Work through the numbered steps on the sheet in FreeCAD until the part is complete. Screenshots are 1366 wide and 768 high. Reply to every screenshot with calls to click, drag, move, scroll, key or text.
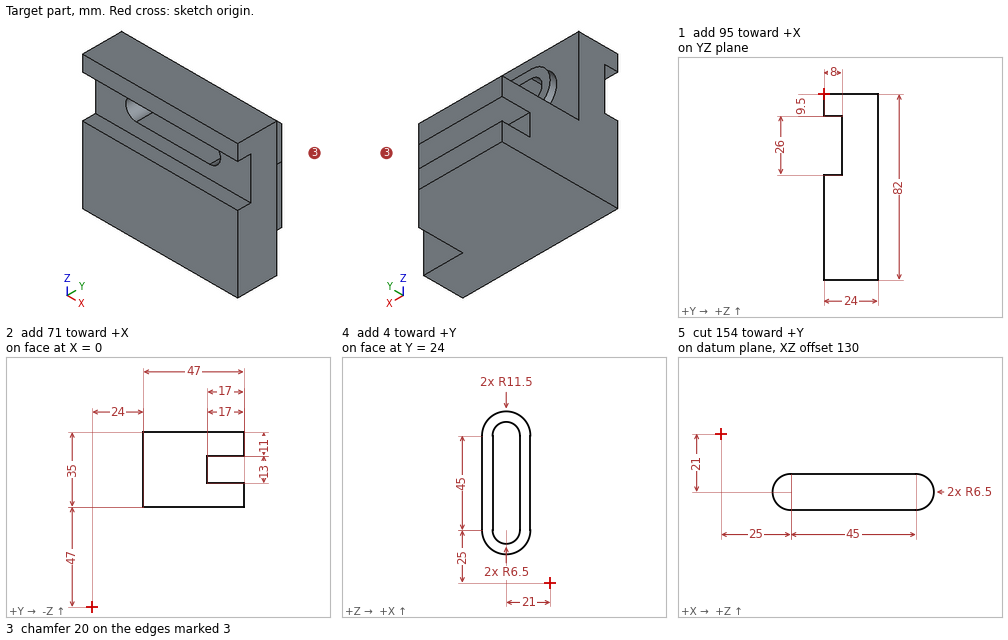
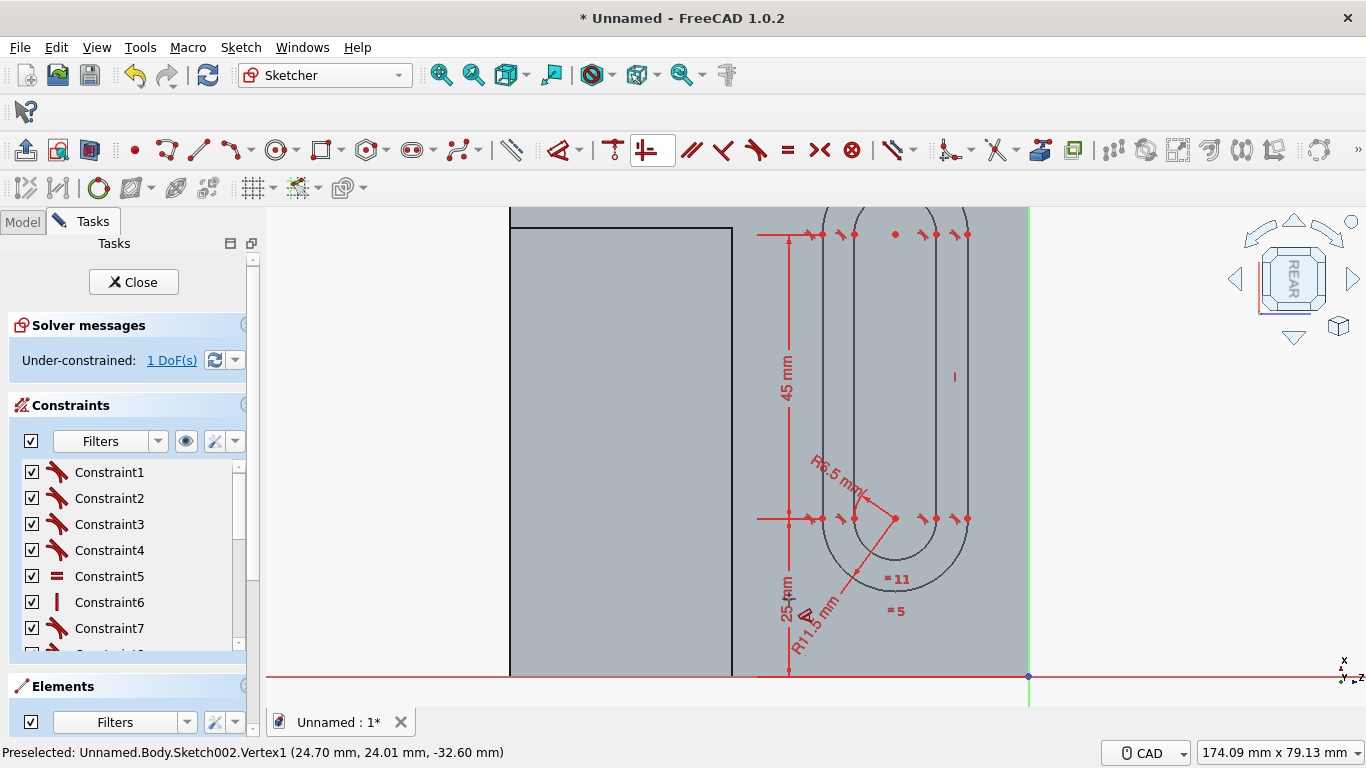
click(895, 519)
click(993, 485)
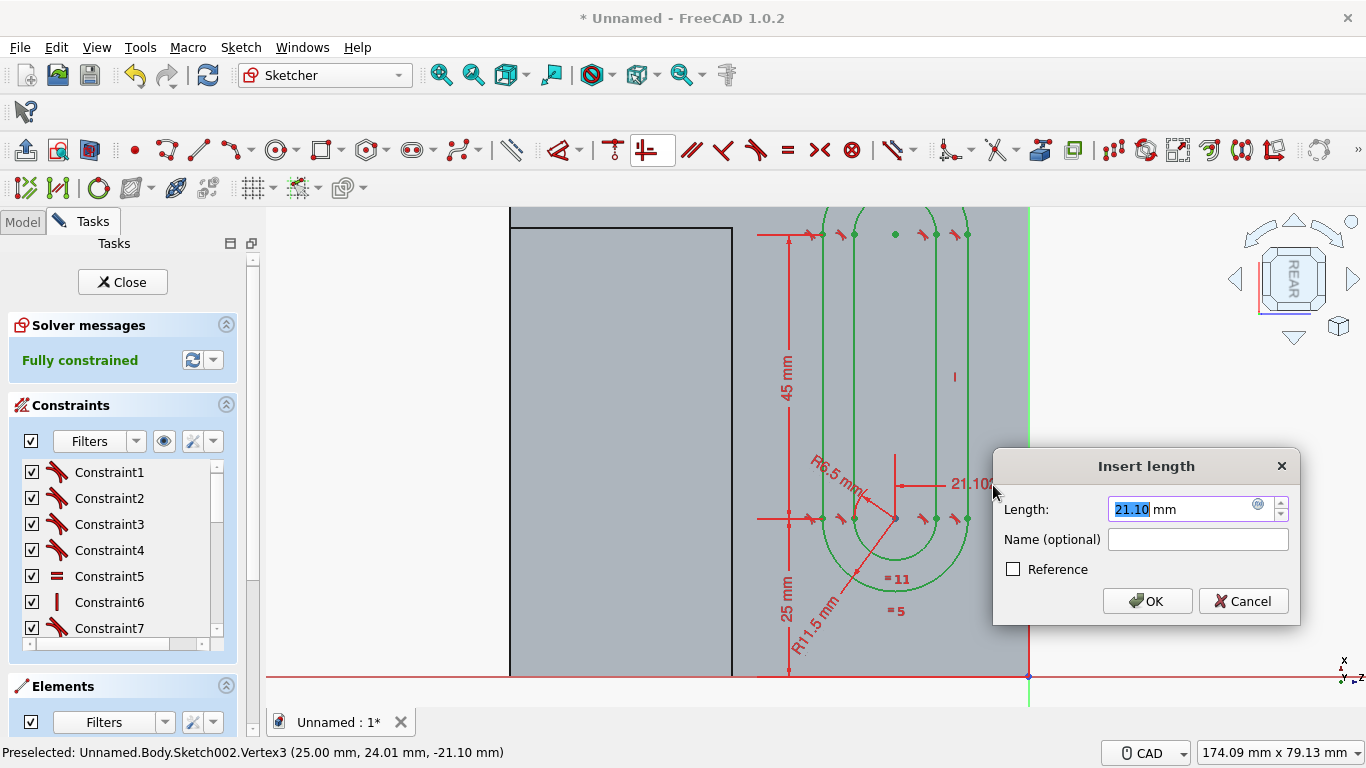
text(21)
key(Return)
key(Escape)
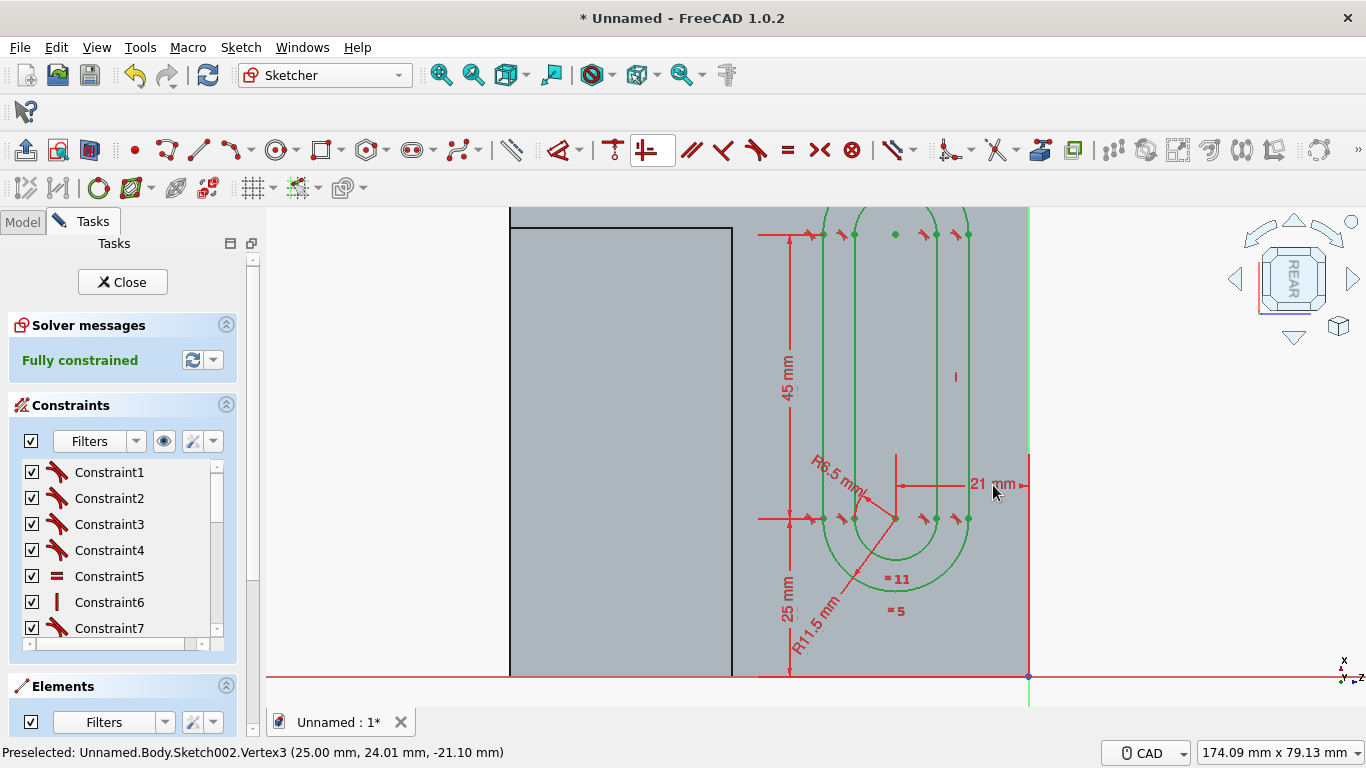
click(123, 282)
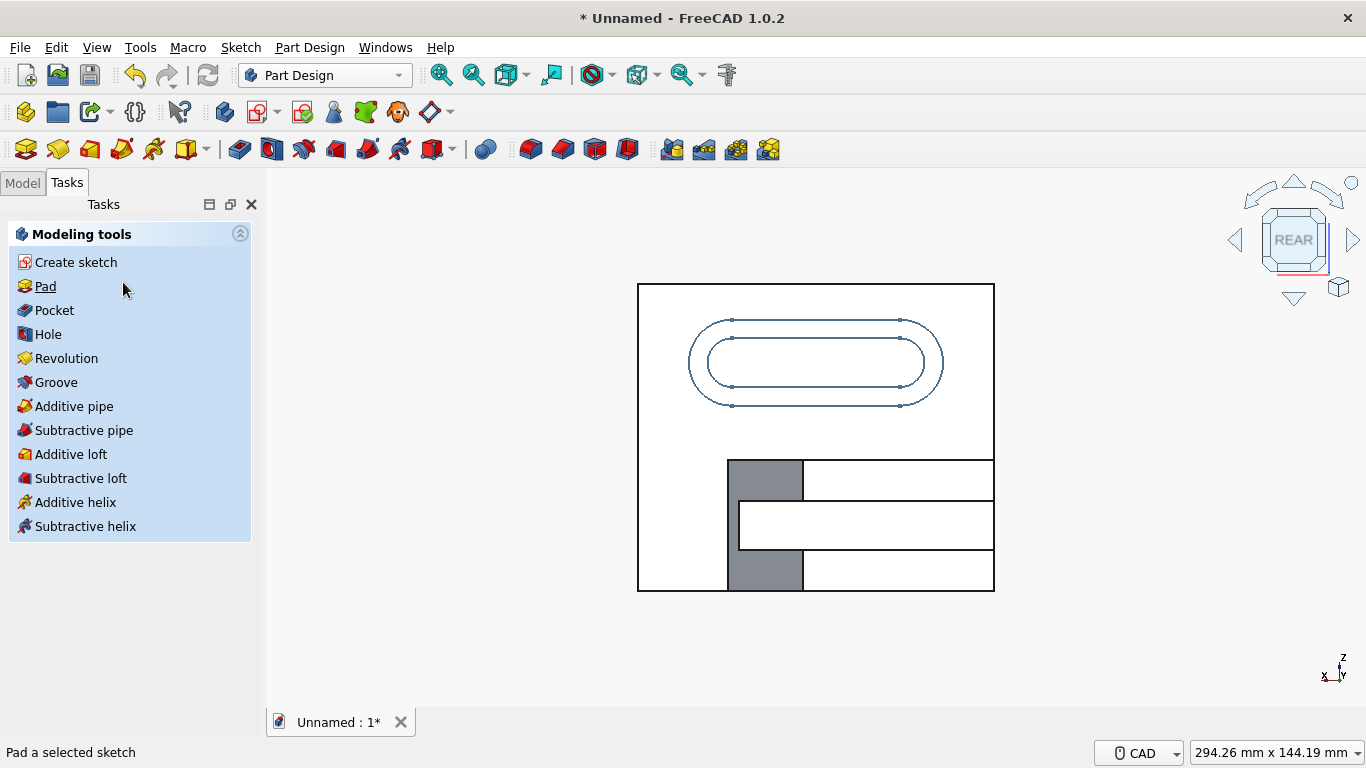
click(26, 150)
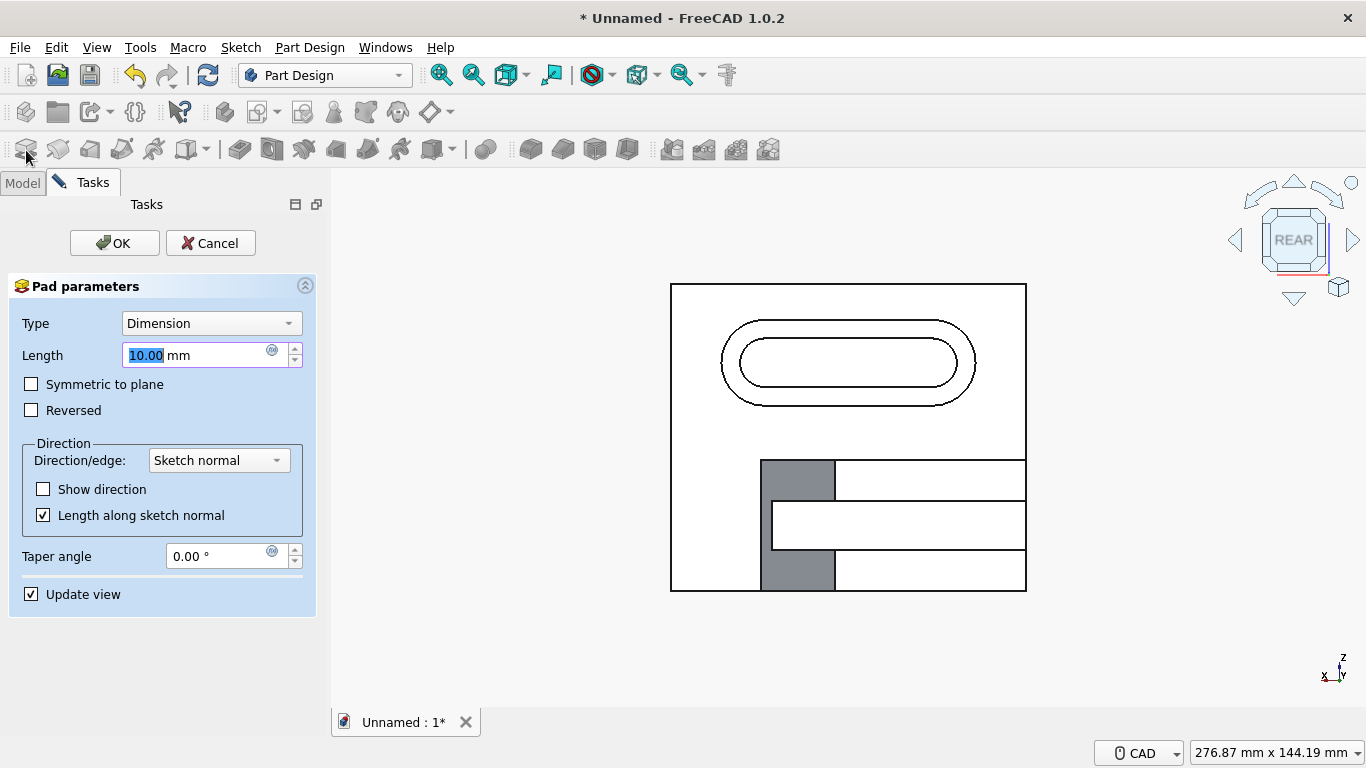
text(4)
key(Tab)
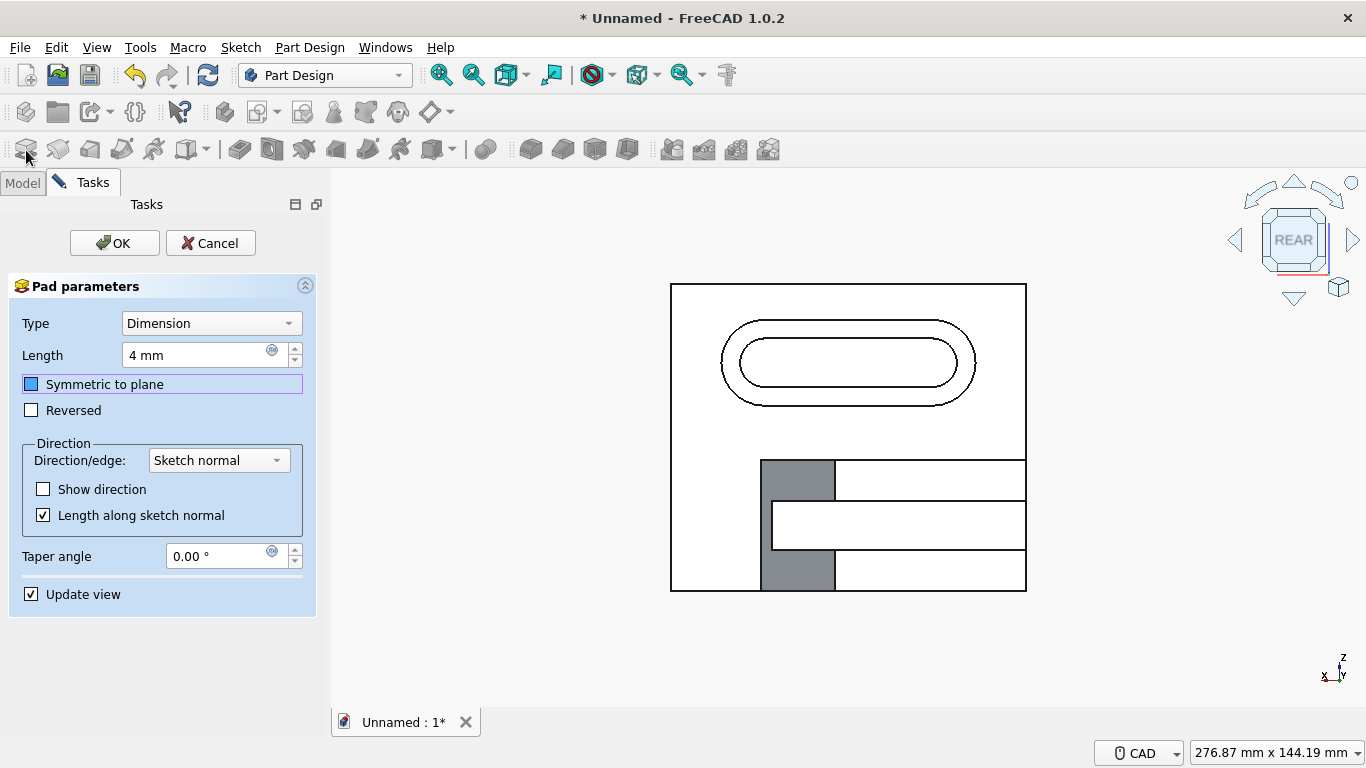
click(115, 243)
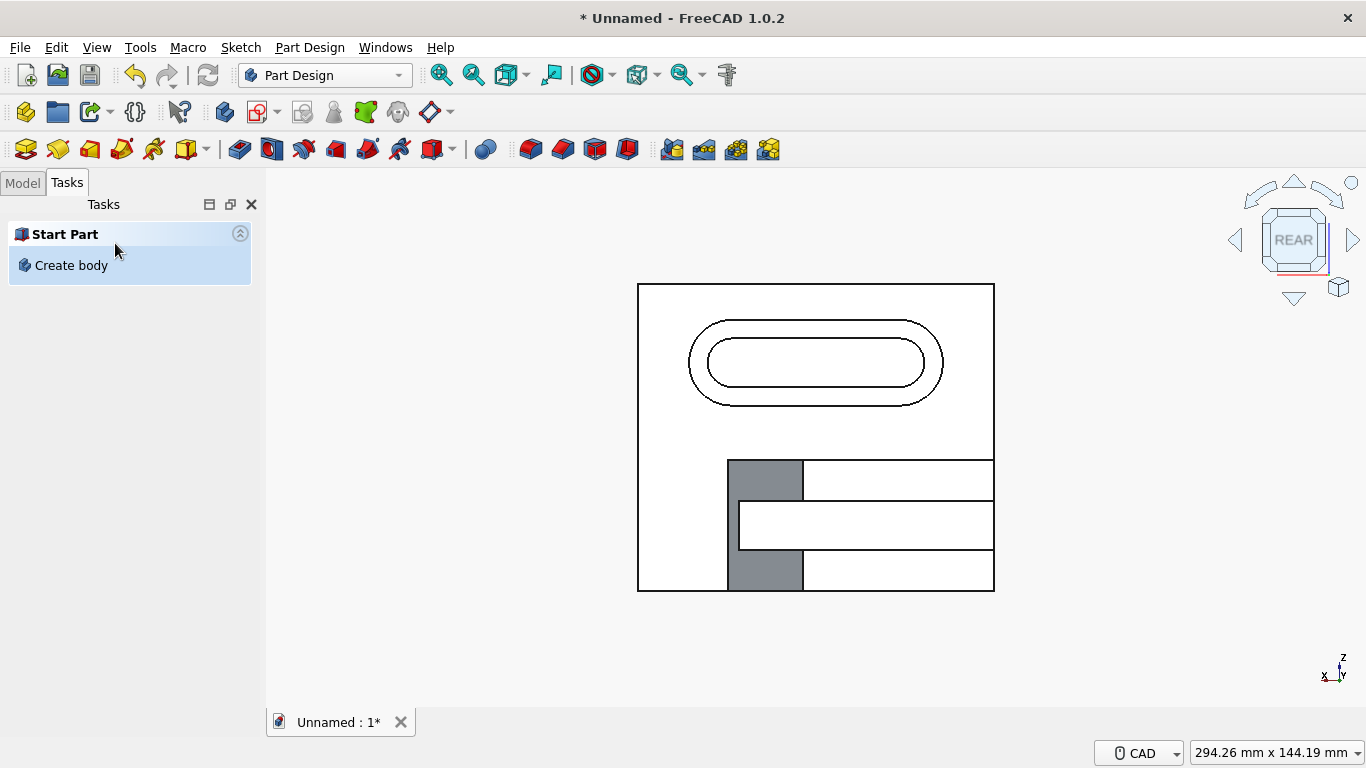
click(23, 182)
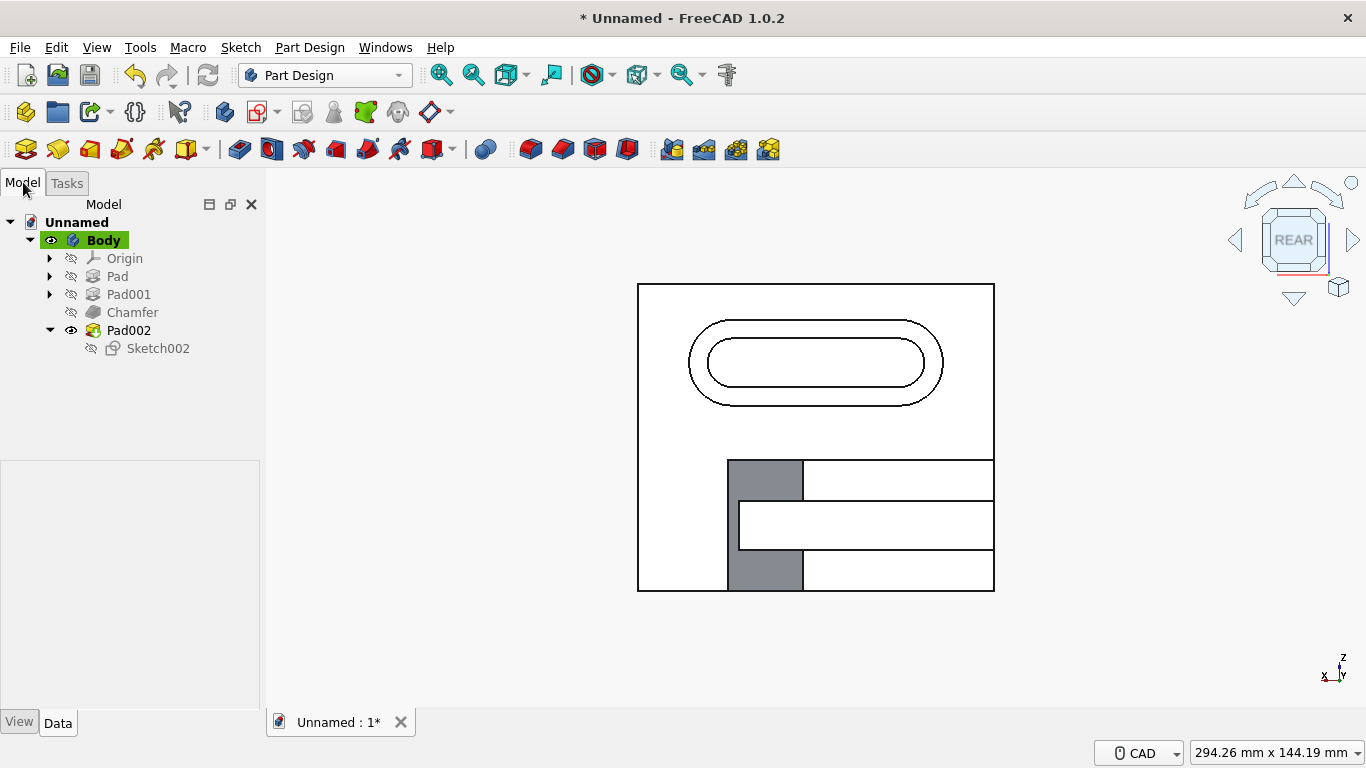
click(50, 258)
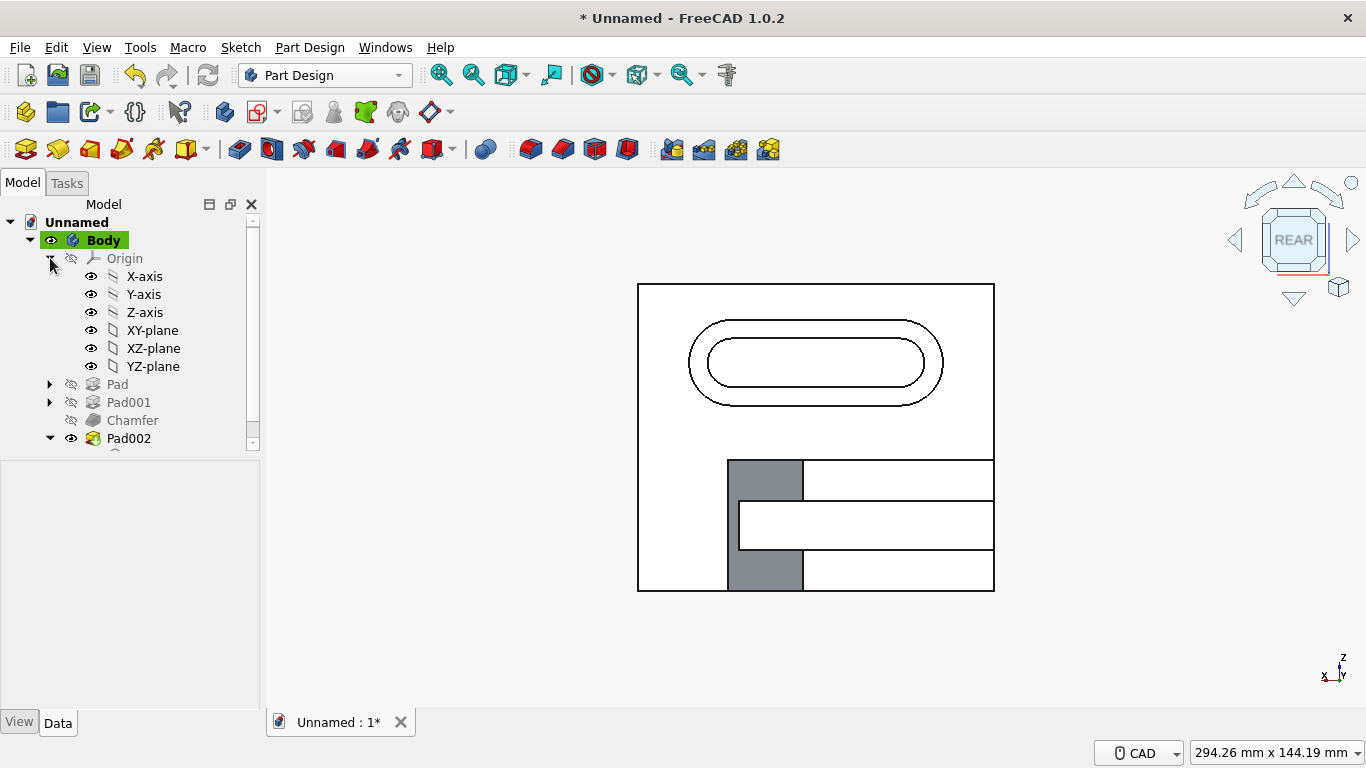
click(136, 348)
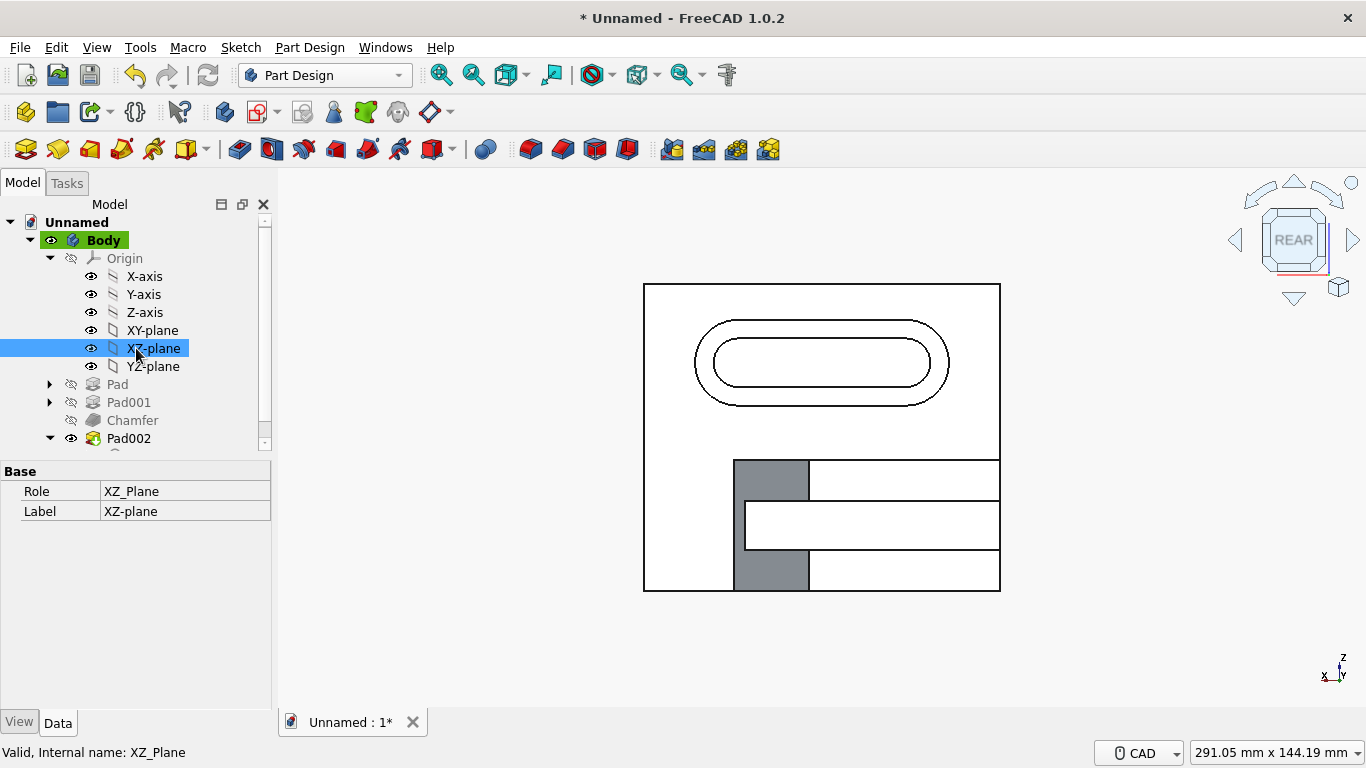
click(430, 112)